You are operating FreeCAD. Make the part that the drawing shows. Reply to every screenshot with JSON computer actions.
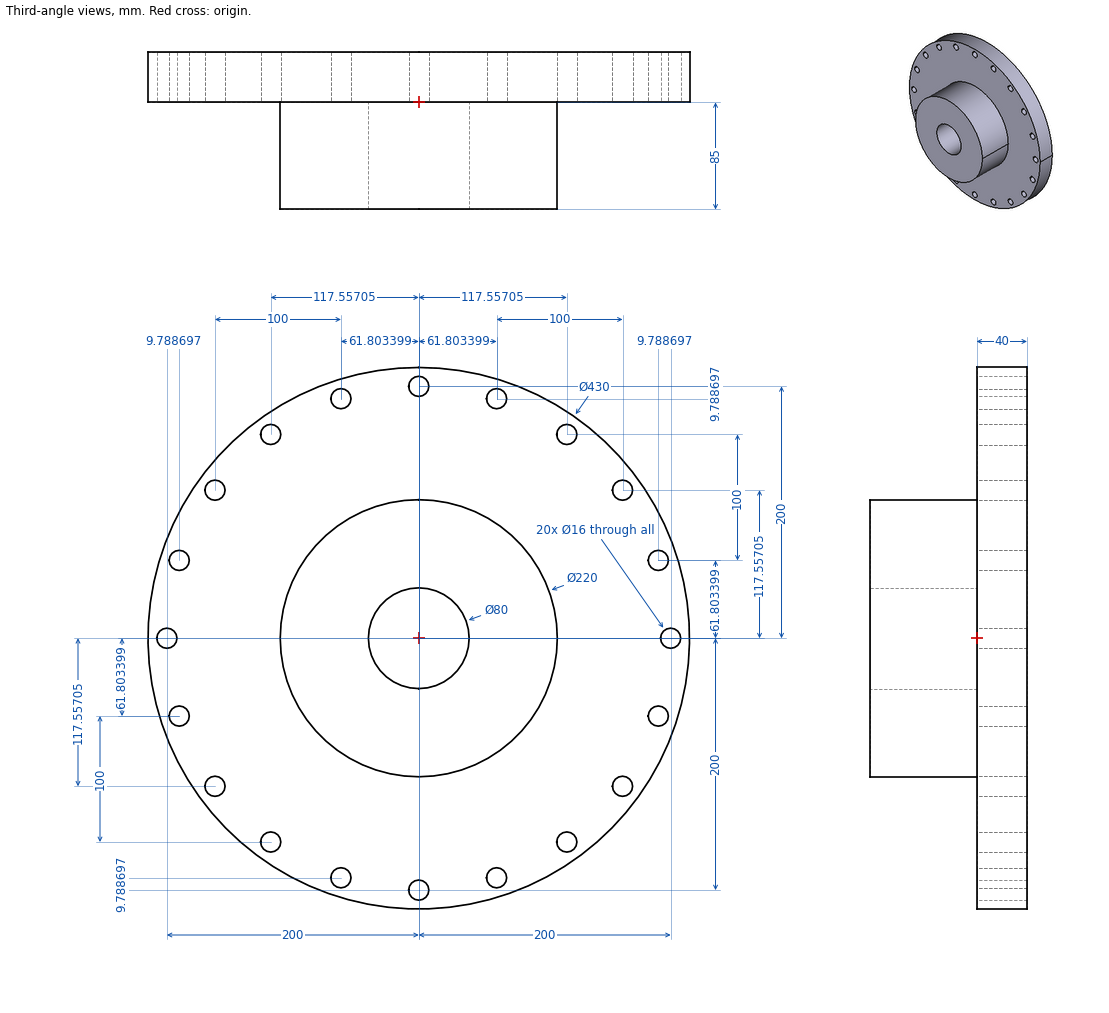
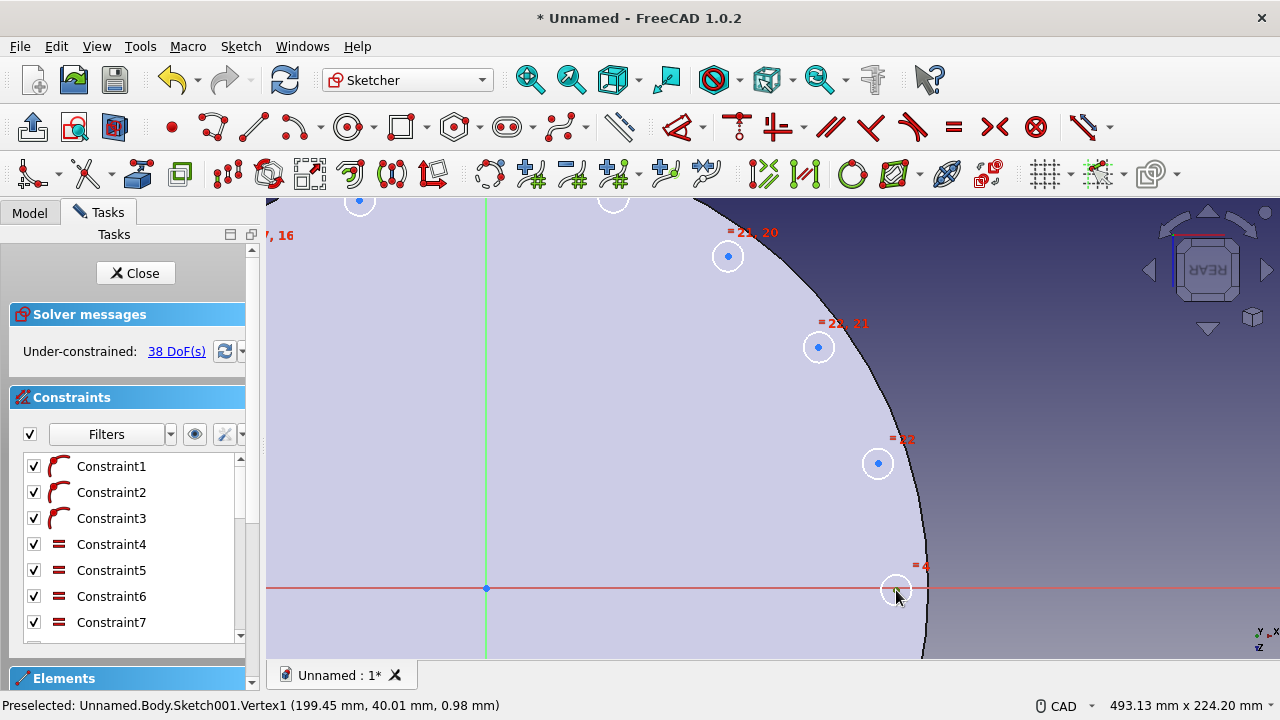
{"action": "left_click", "coordinate": [353, 588]}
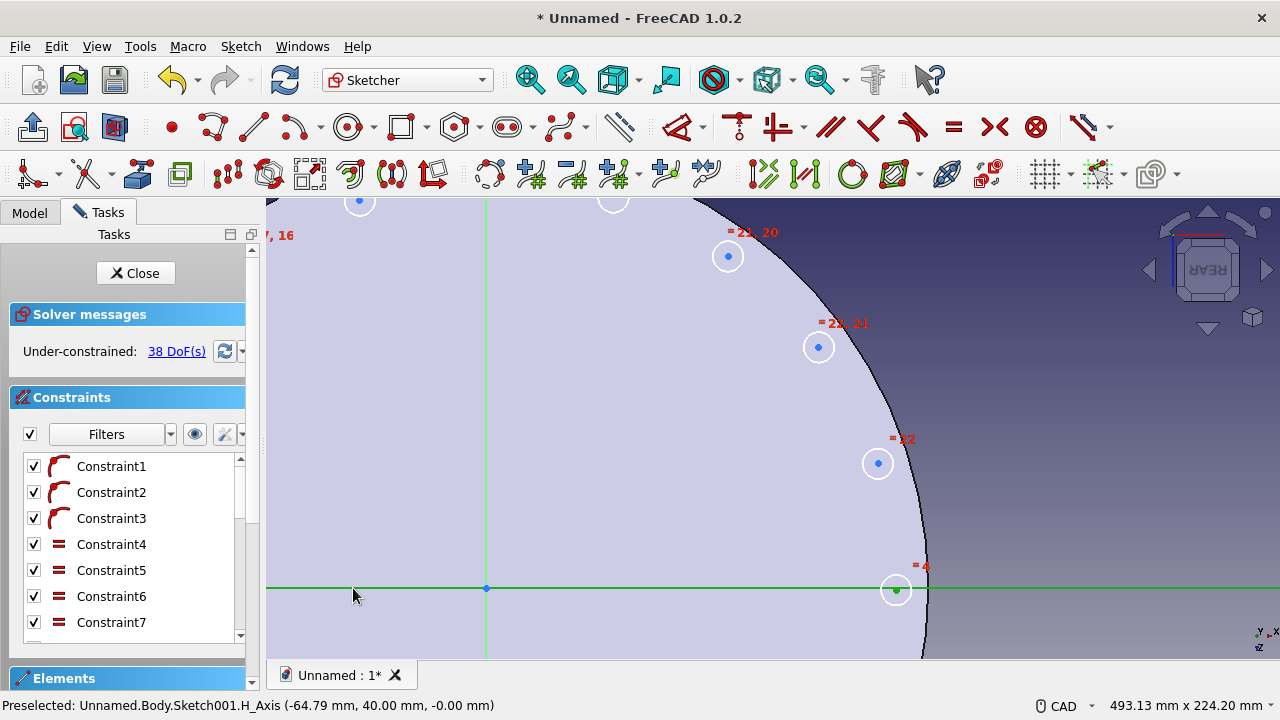
{"action": "left_click", "coordinate": [737, 128]}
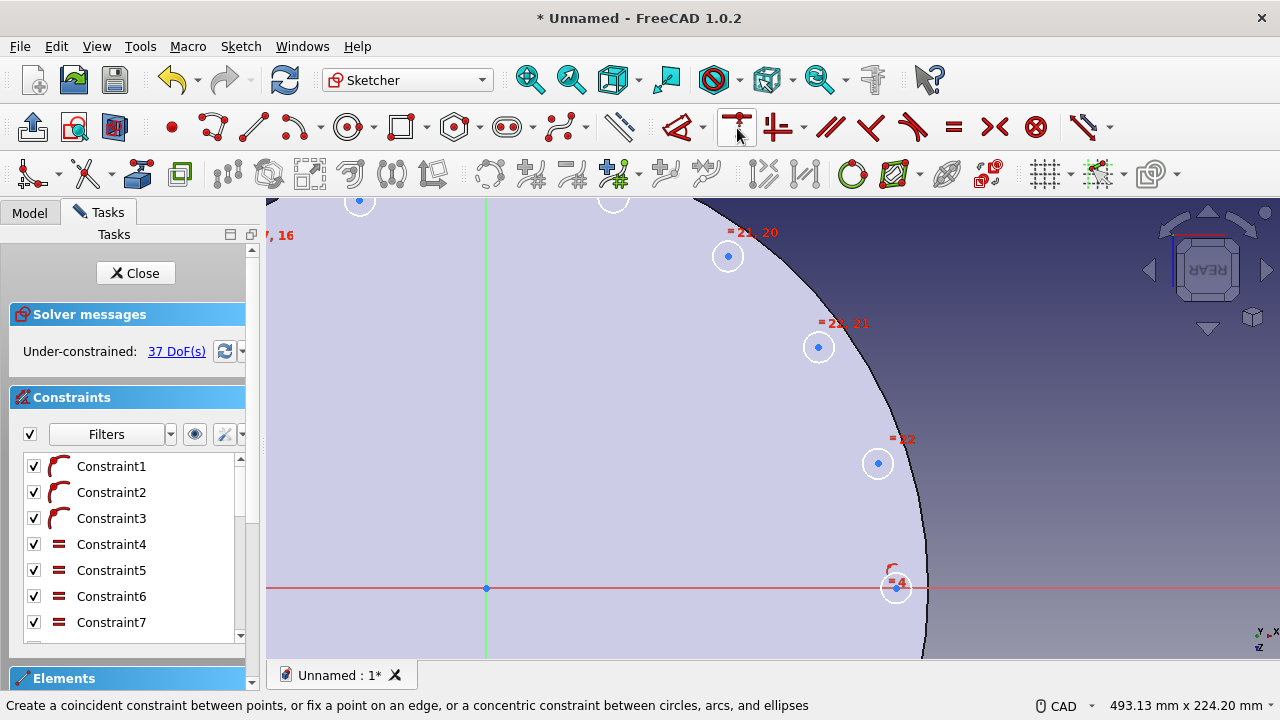
{"action": "scroll", "coordinate": [832, 336], "scroll_direction": "down", "scroll_amount": 5}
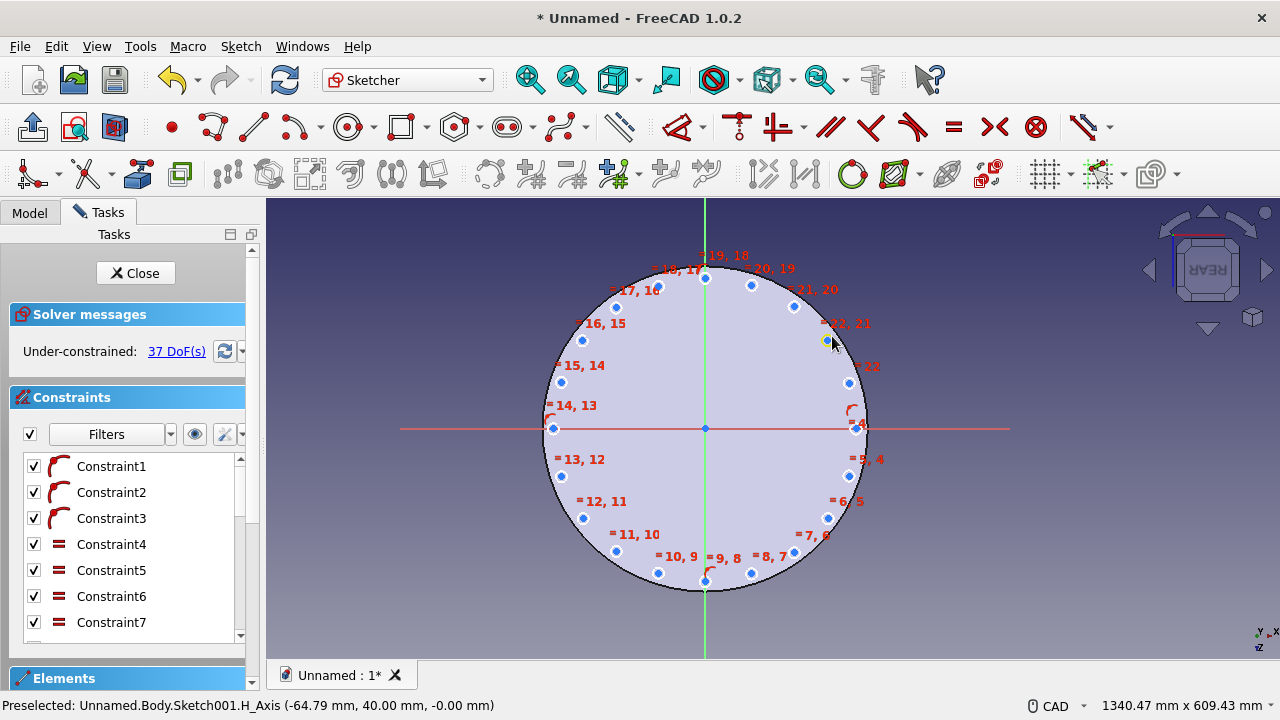
{"action": "left_click", "coordinate": [752, 574]}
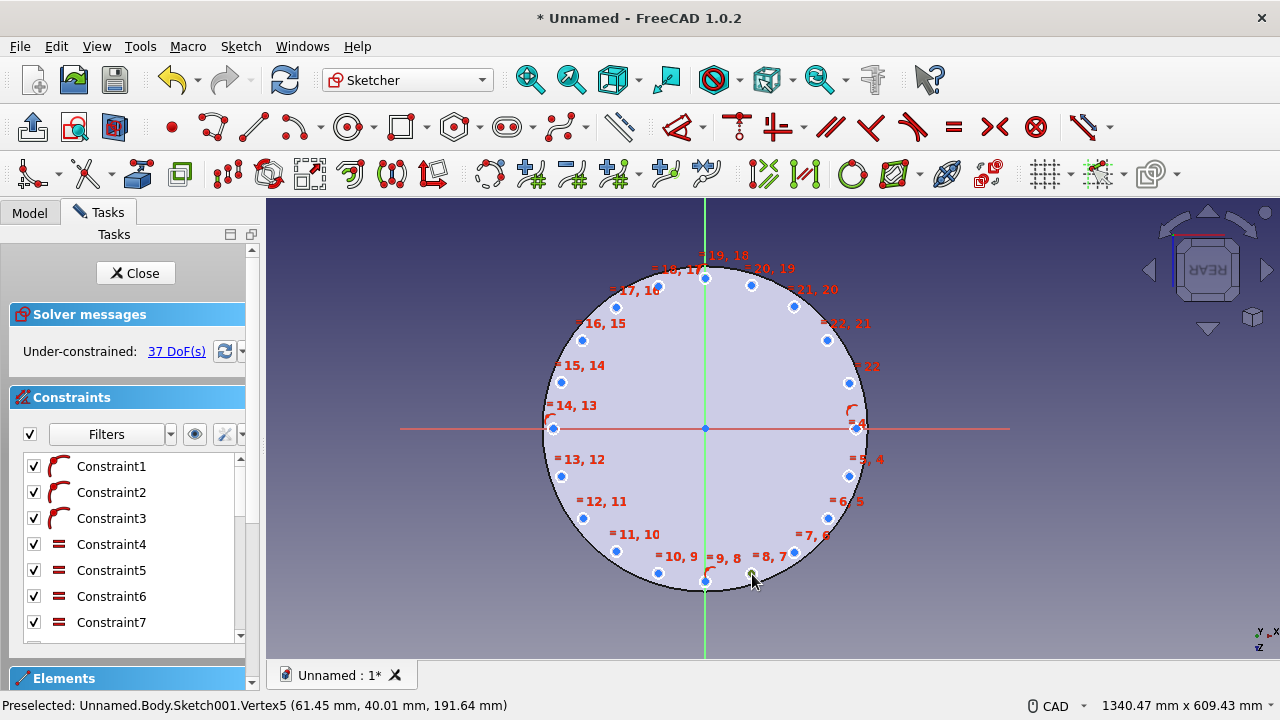
{"action": "left_click", "coordinate": [658, 573]}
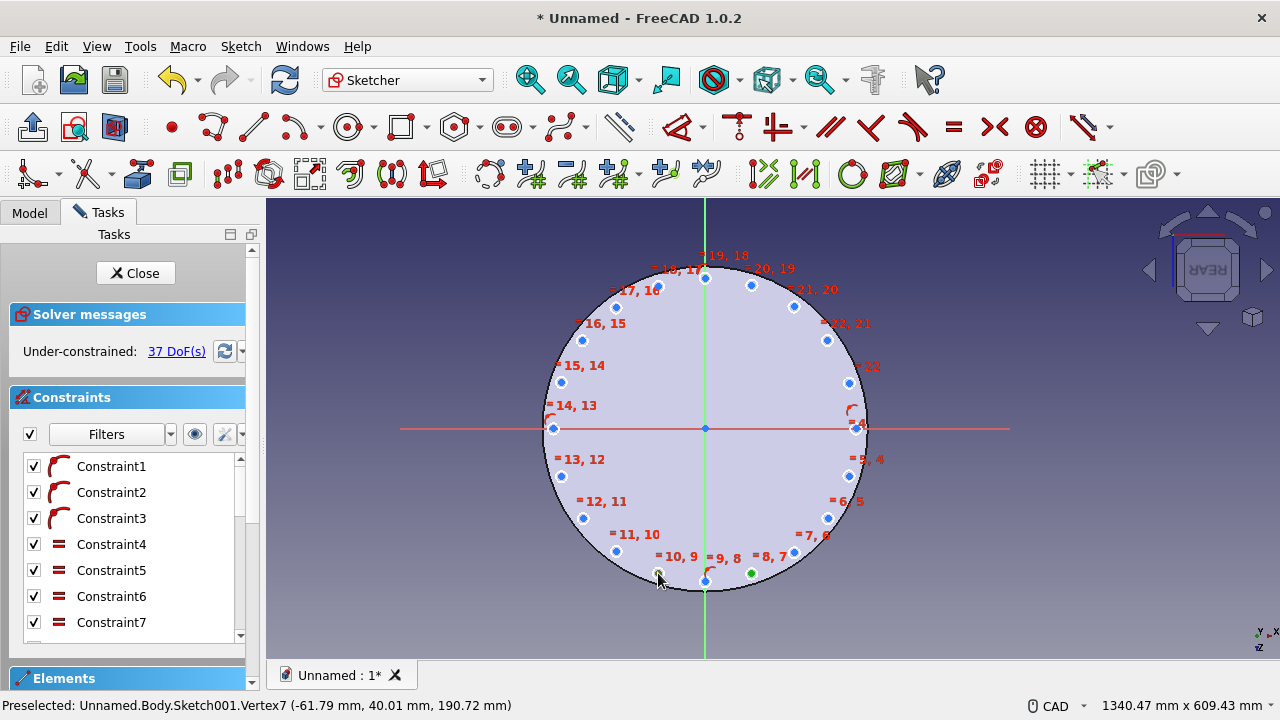
{"action": "left_click", "coordinate": [804, 128]}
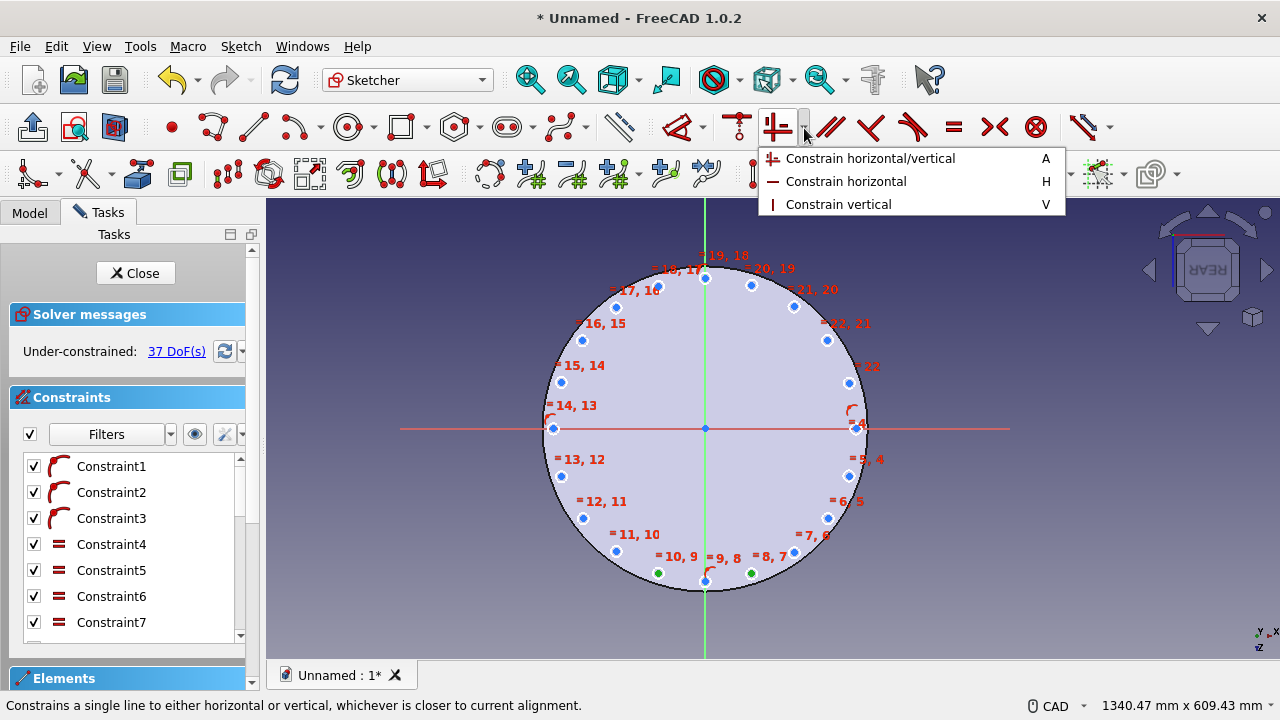
{"action": "left_click", "coordinate": [912, 182]}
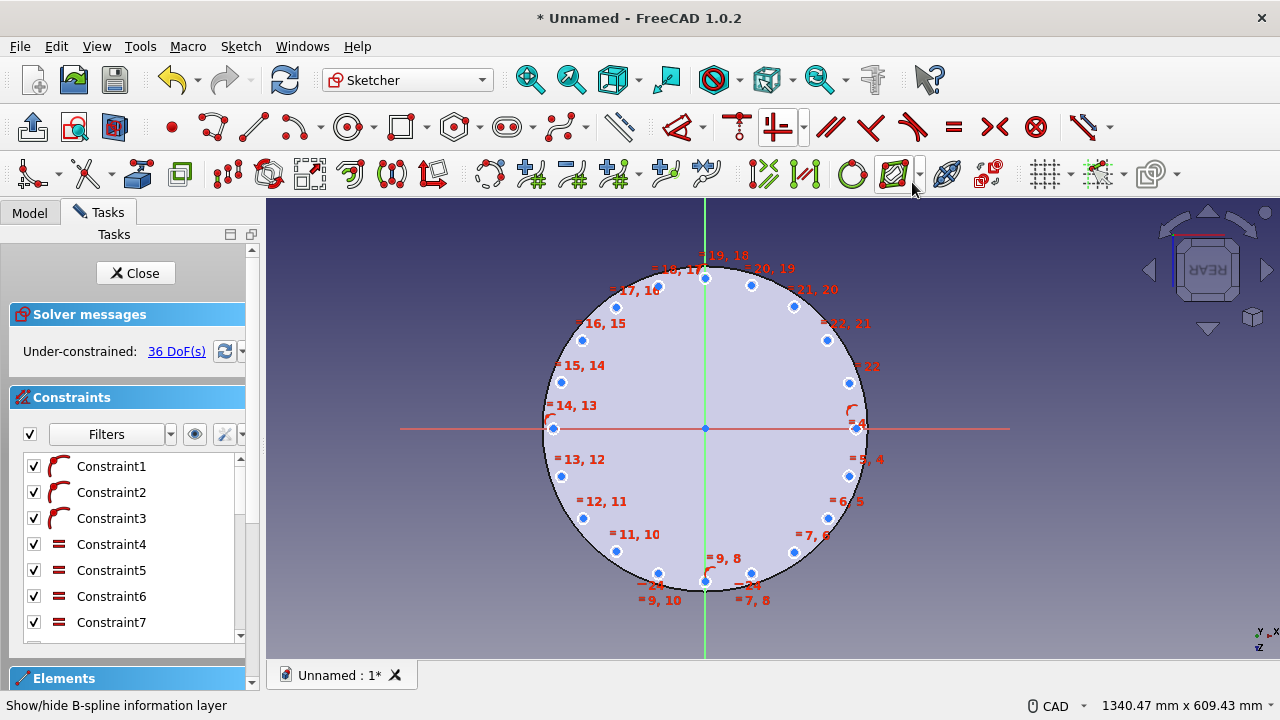
{"action": "left_click", "coordinate": [794, 553]}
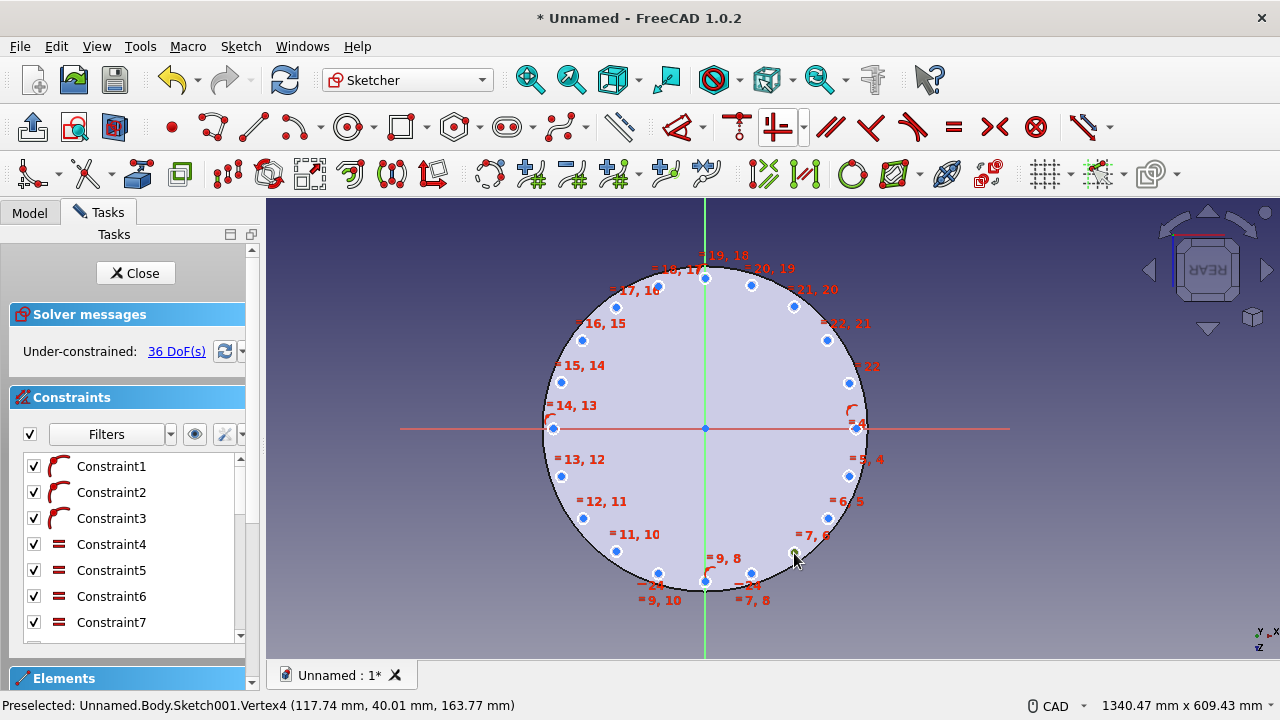
{"action": "left_click", "coordinate": [616, 552]}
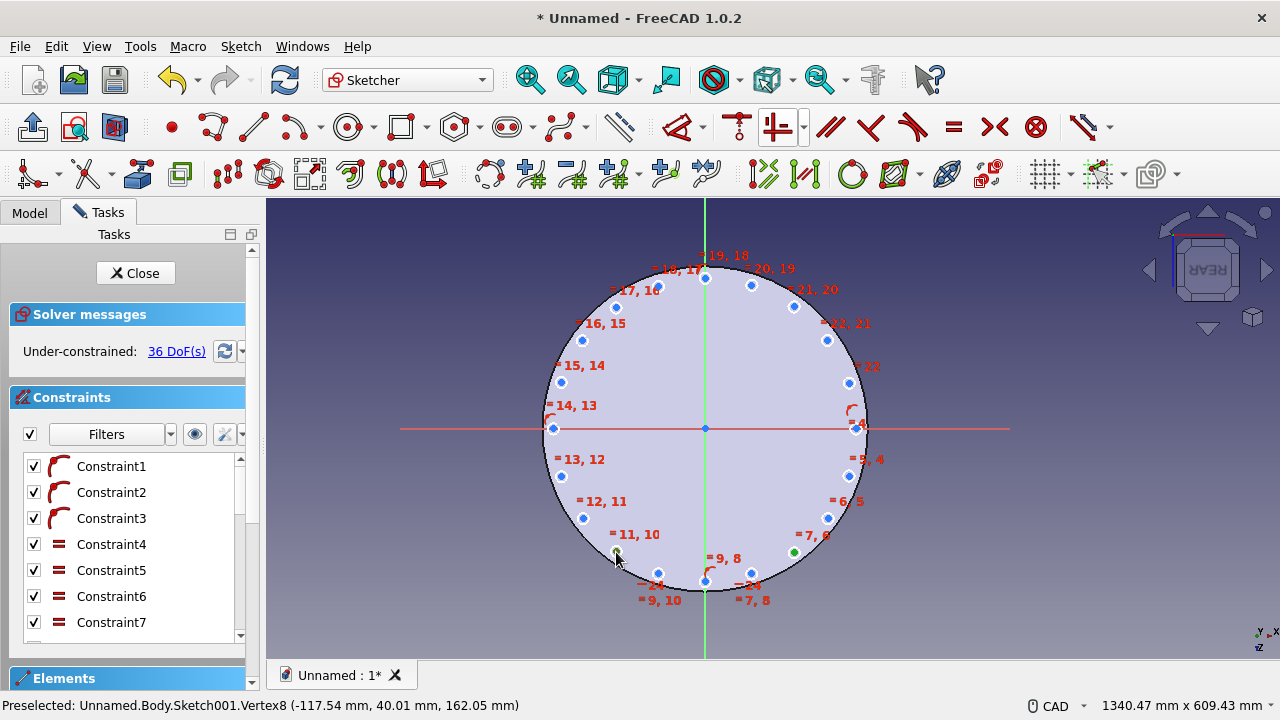
{"action": "key", "text": "h"}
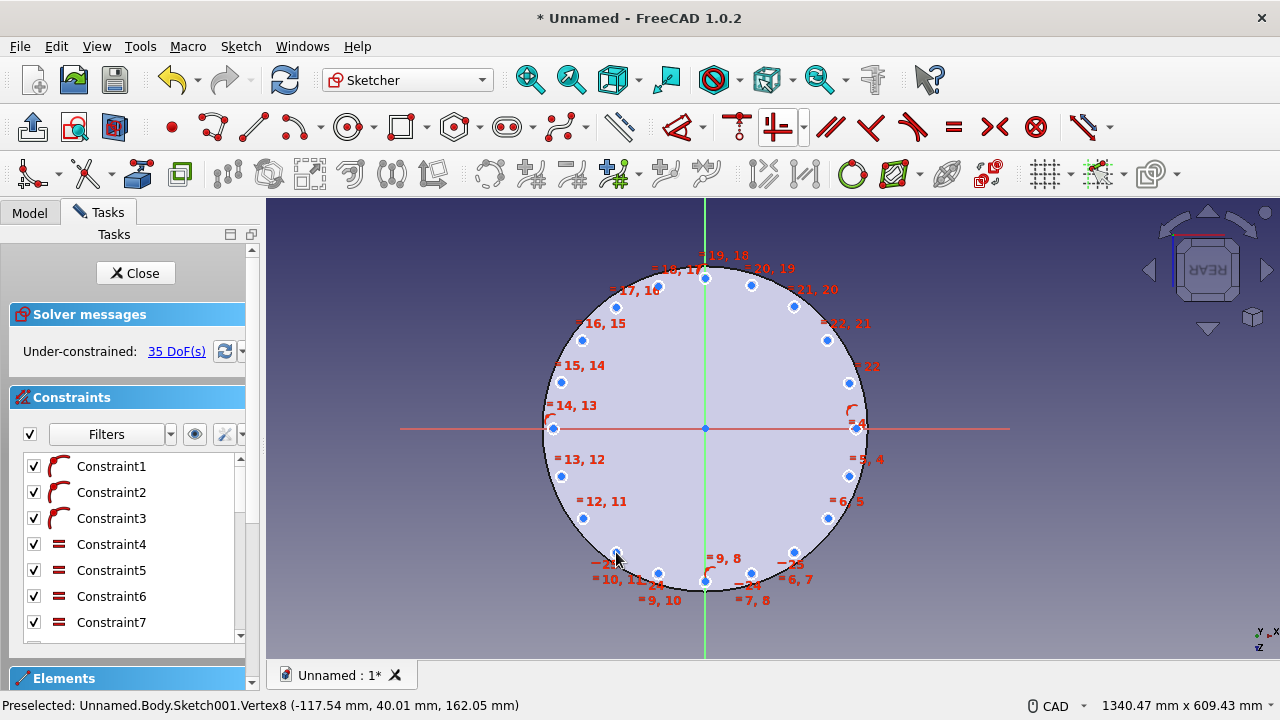
{"action": "left_click", "coordinate": [828, 519]}